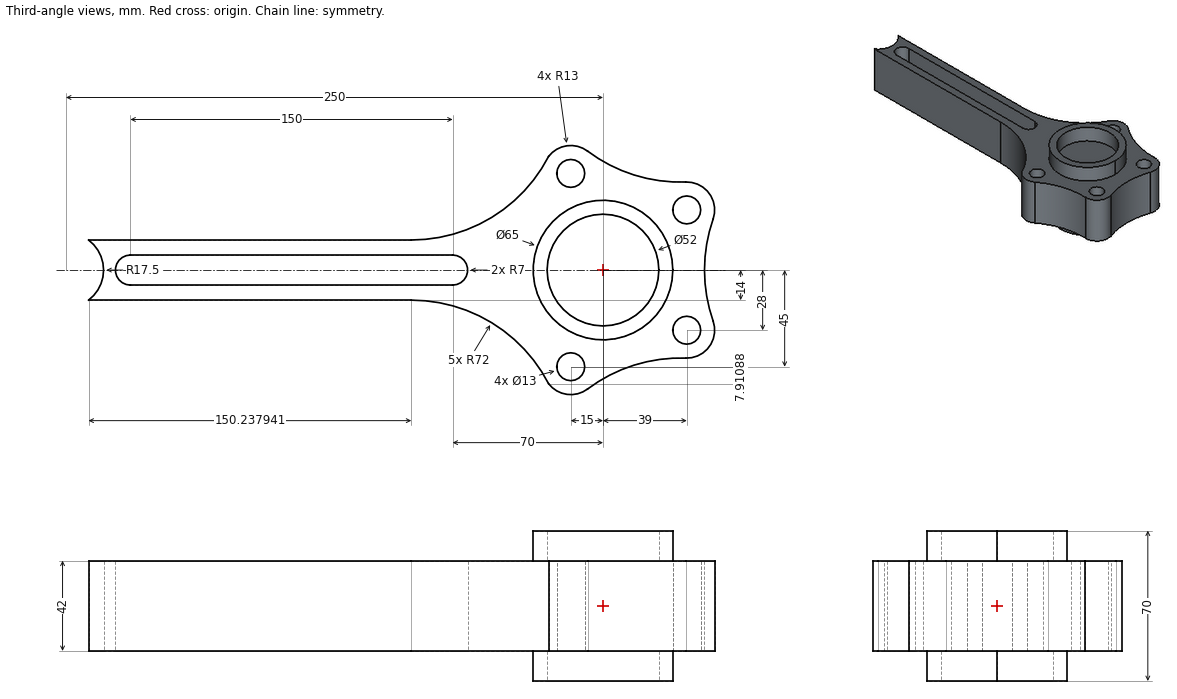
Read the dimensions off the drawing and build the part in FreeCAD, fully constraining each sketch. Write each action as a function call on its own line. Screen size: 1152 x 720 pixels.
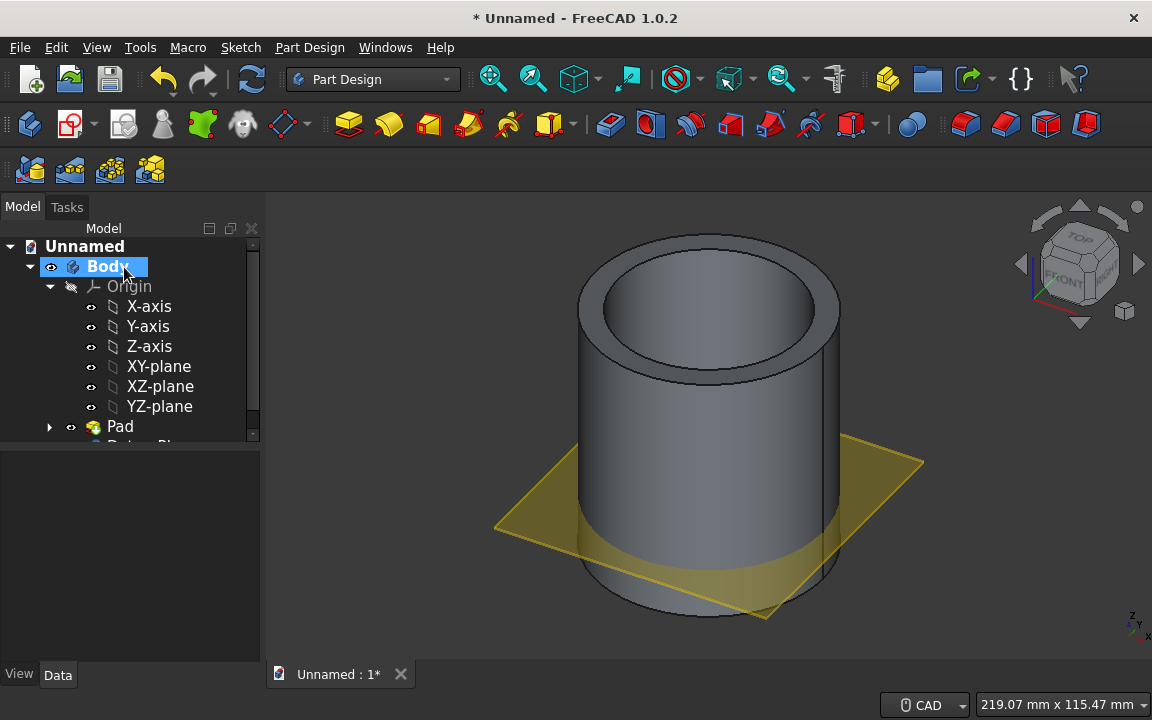
scroll(100, 342, down, 3)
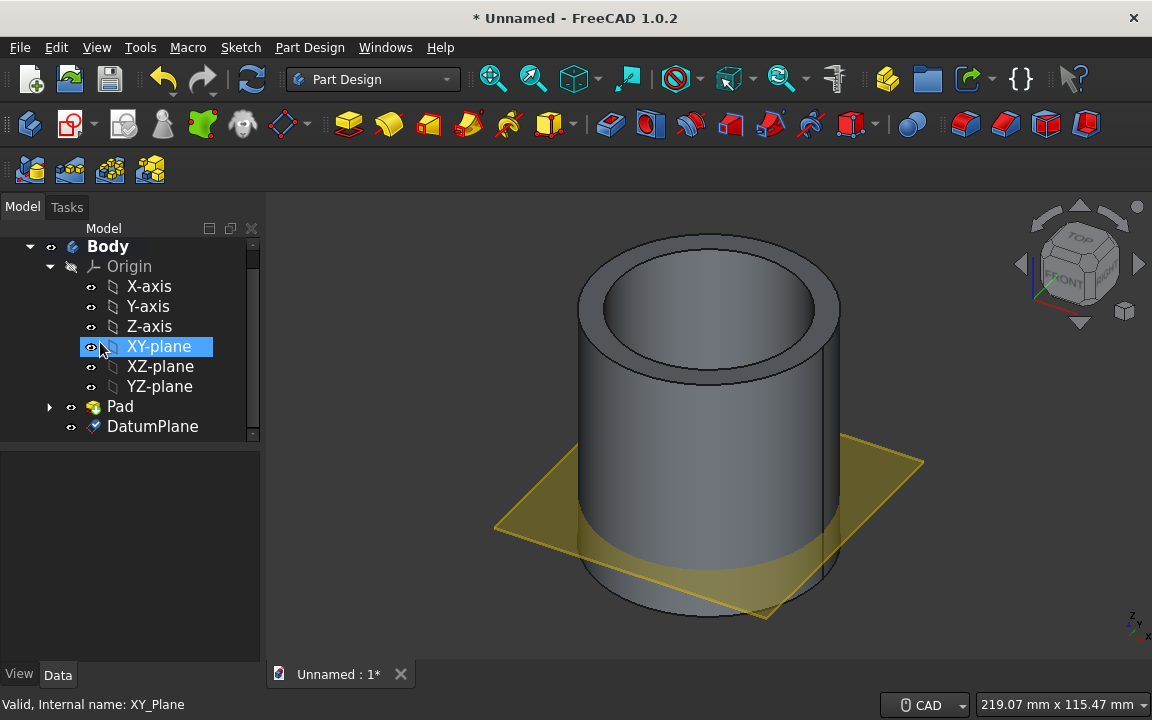
click(116, 427)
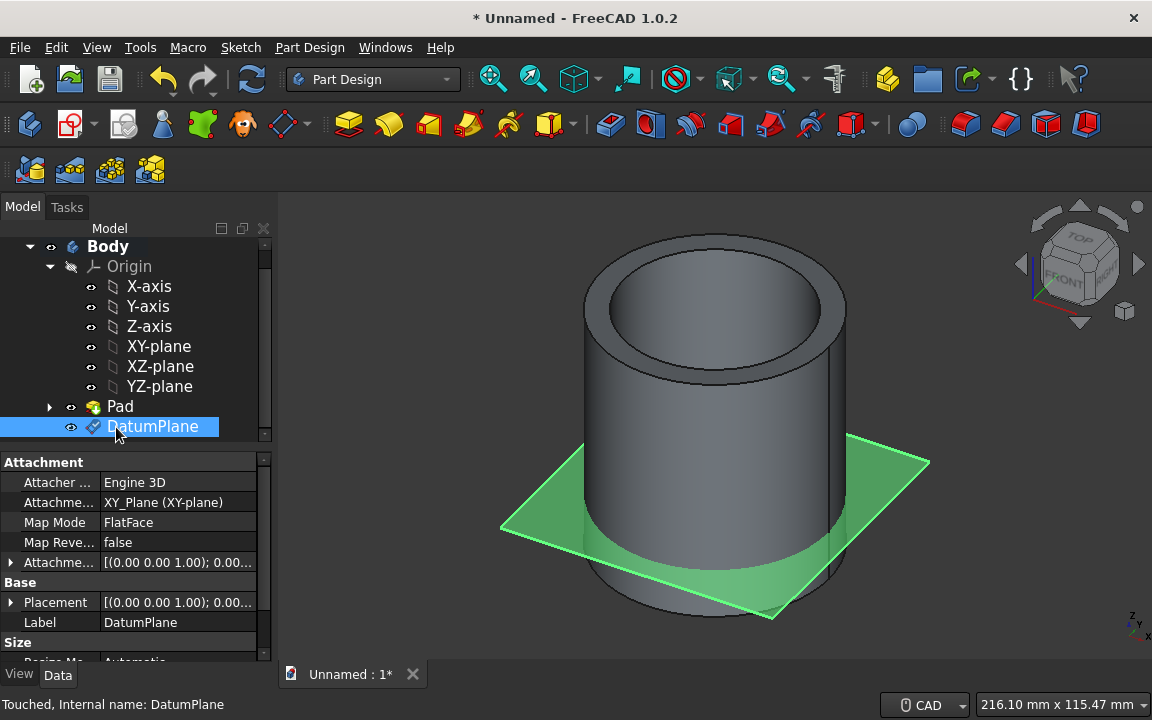
click(70, 124)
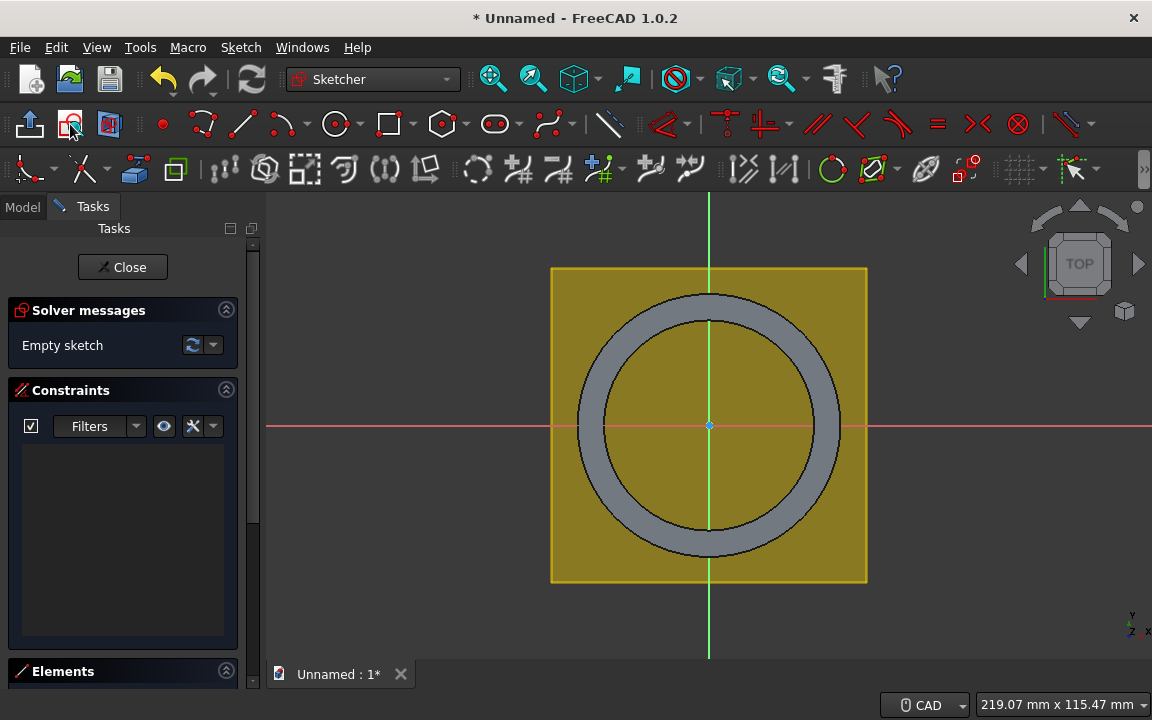
click(110, 124)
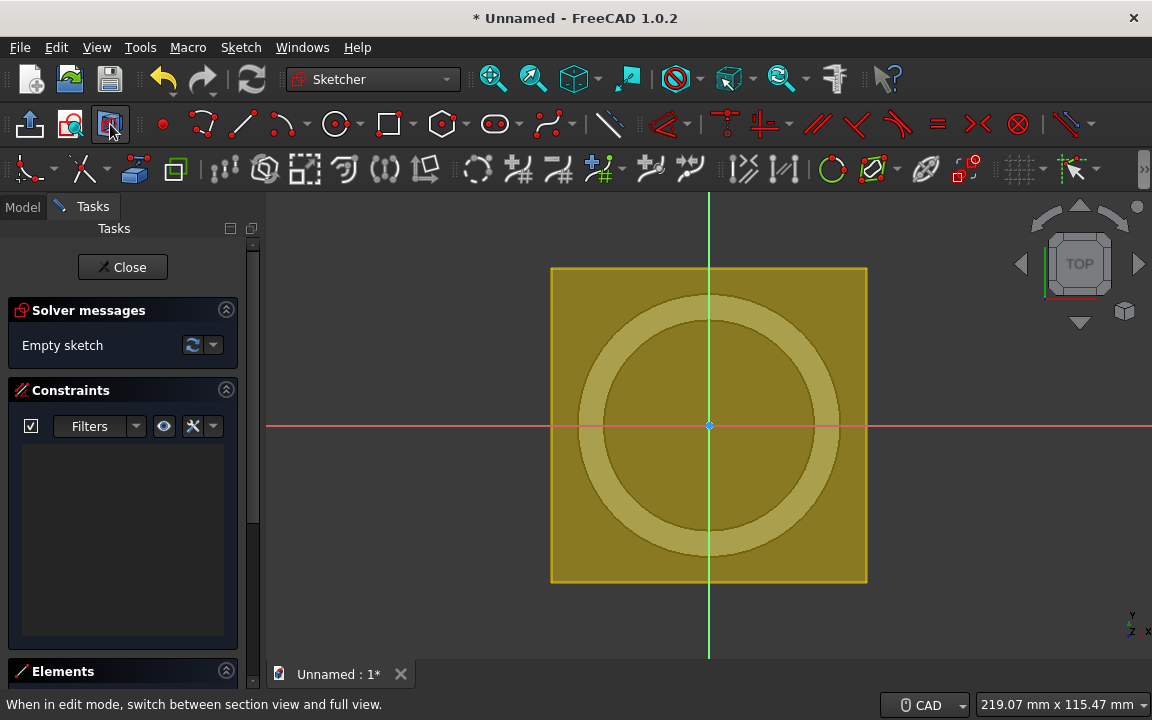
scroll(895, 426, down, 4)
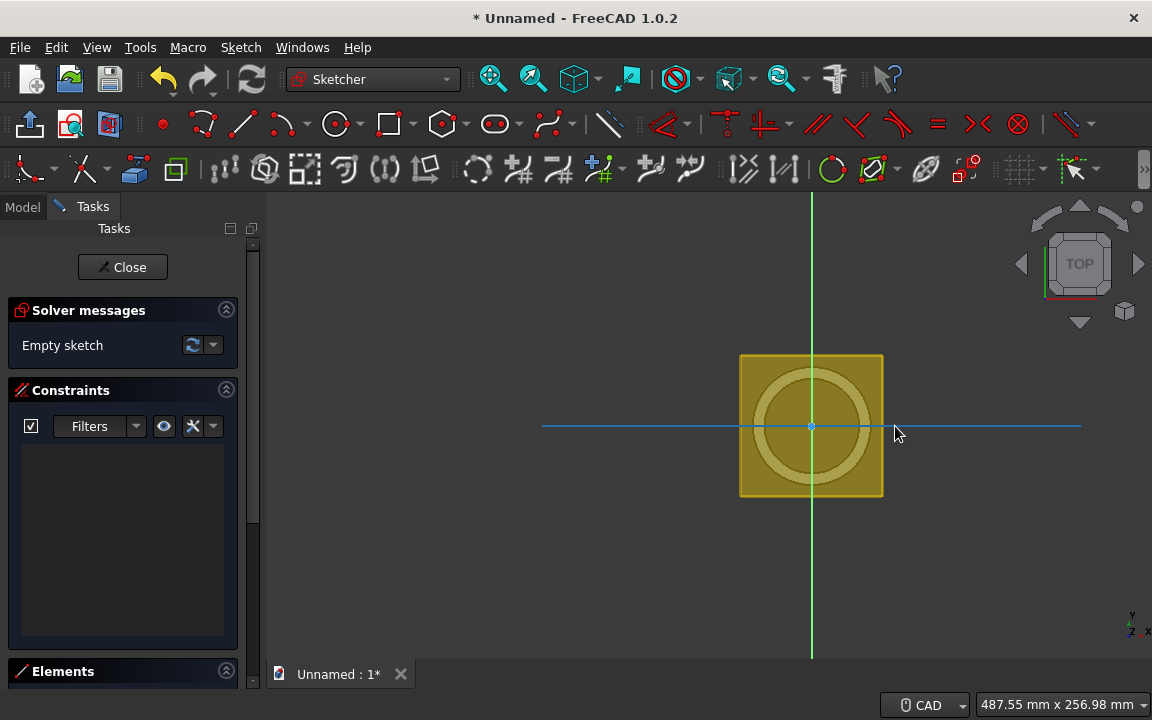
click(244, 124)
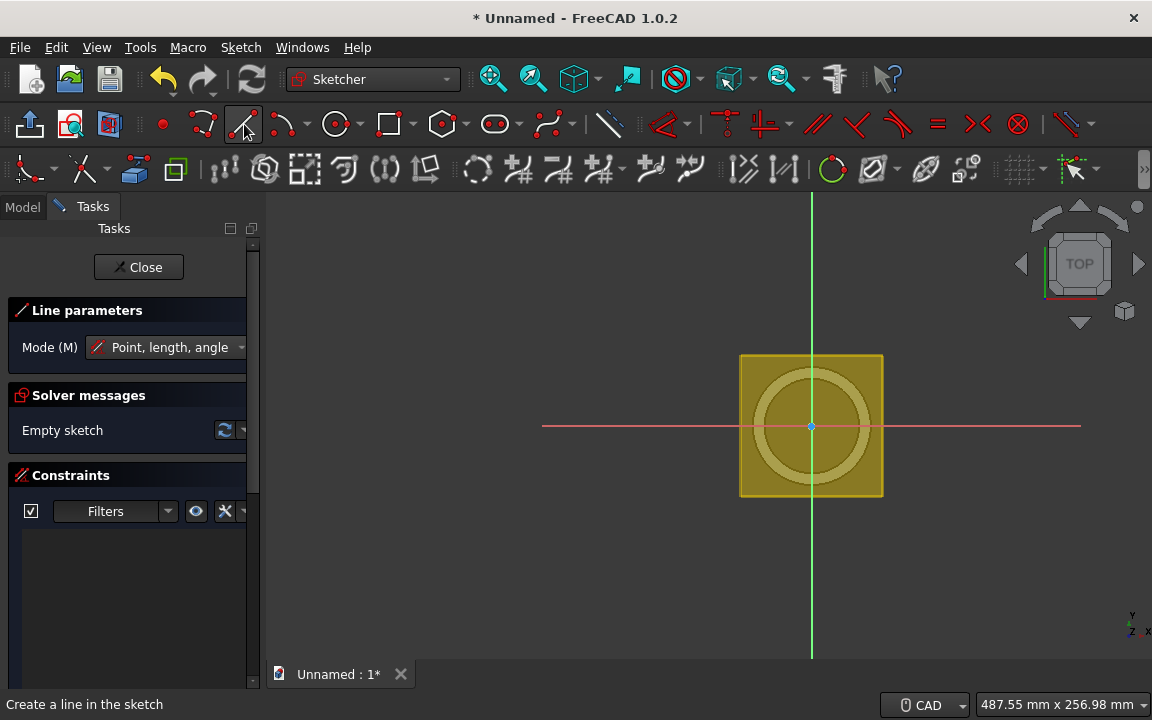
click(650, 451)
click(377, 451)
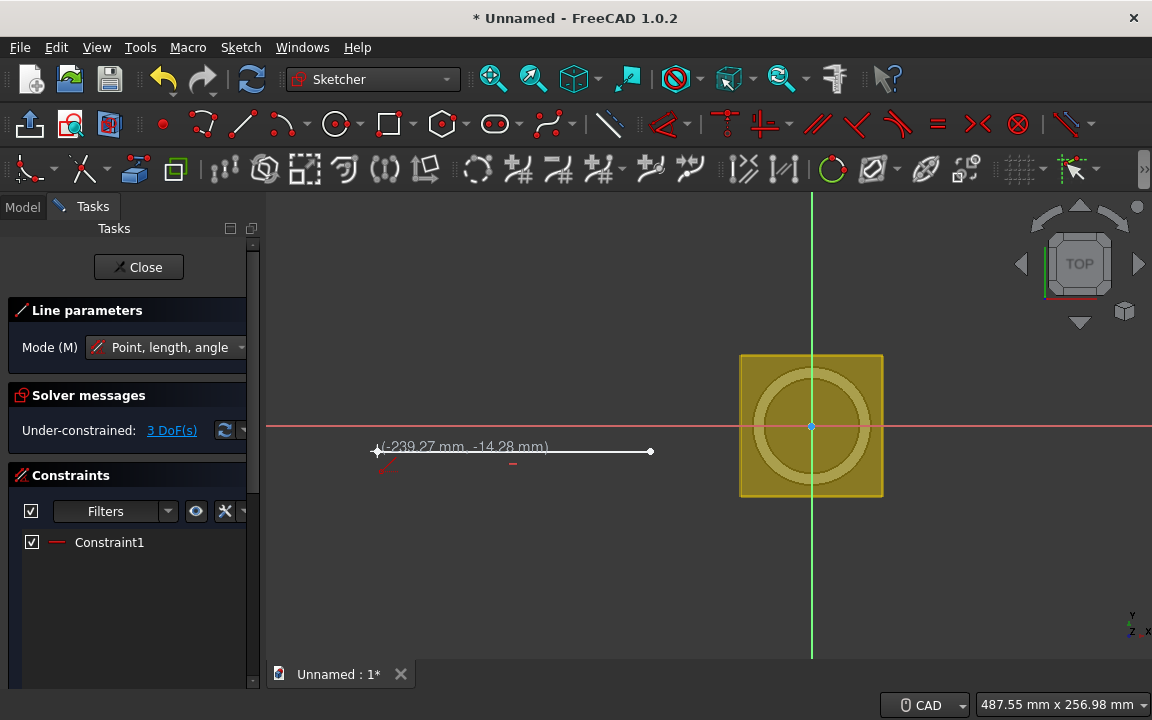
click(377, 401)
click(650, 401)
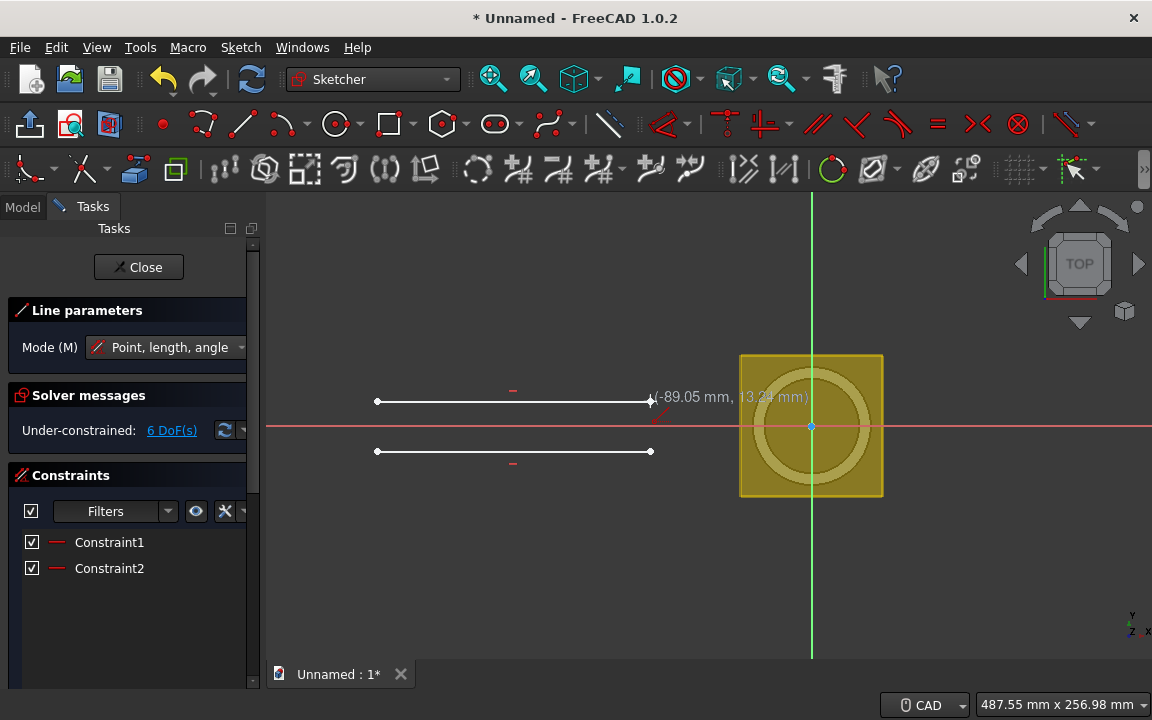
click(310, 124)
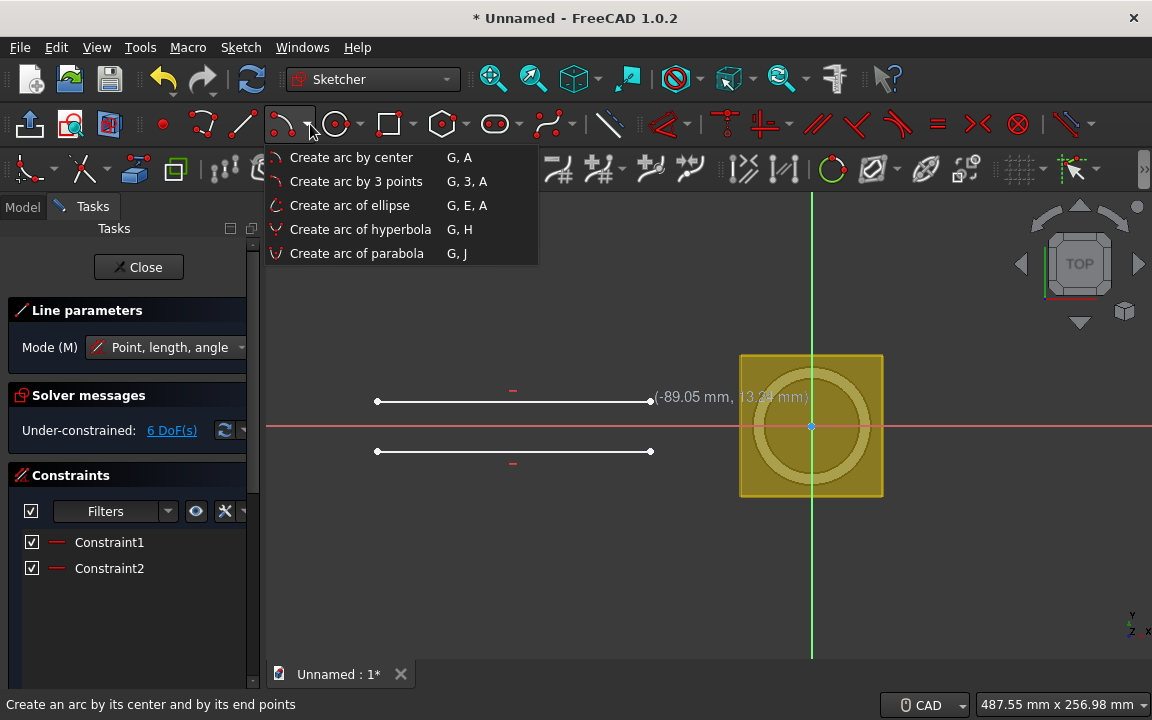
click(402, 181)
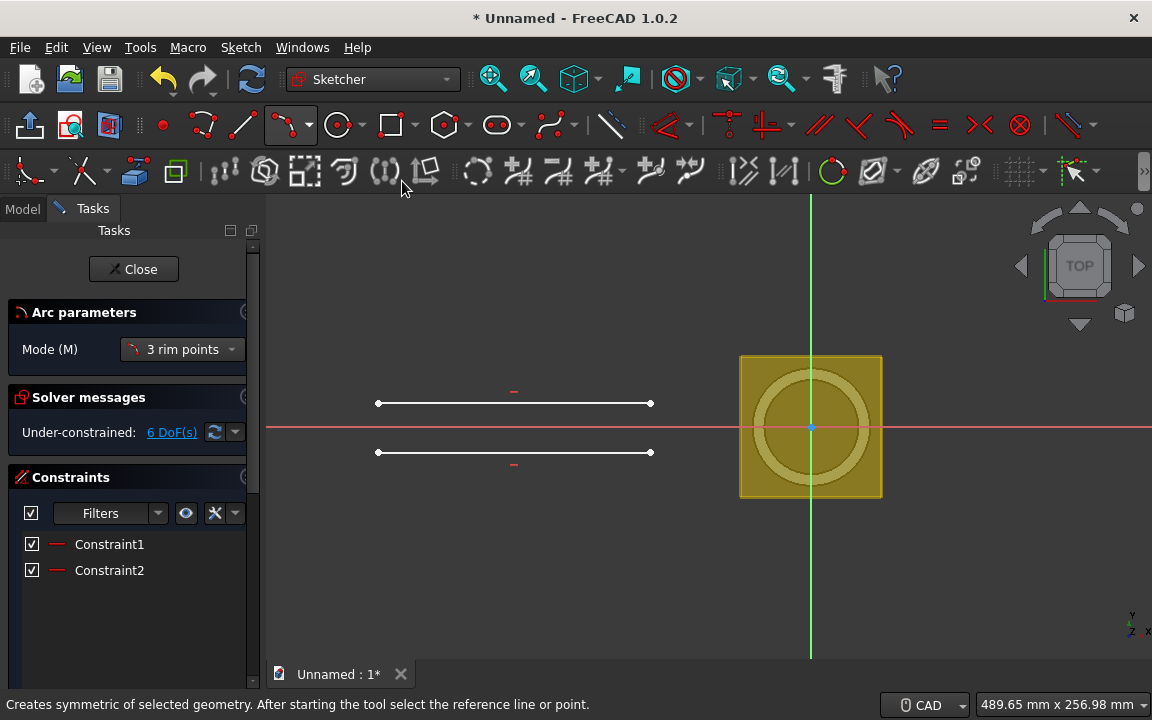
click(378, 453)
click(378, 403)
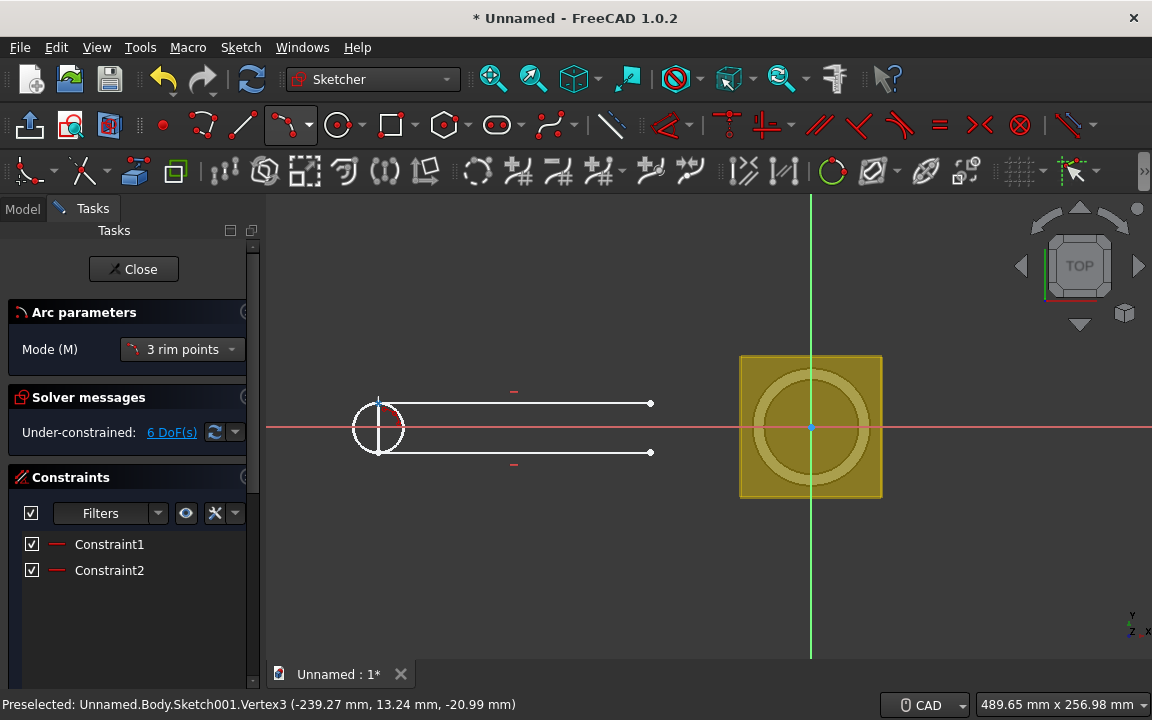
scroll(389, 439, up, 3)